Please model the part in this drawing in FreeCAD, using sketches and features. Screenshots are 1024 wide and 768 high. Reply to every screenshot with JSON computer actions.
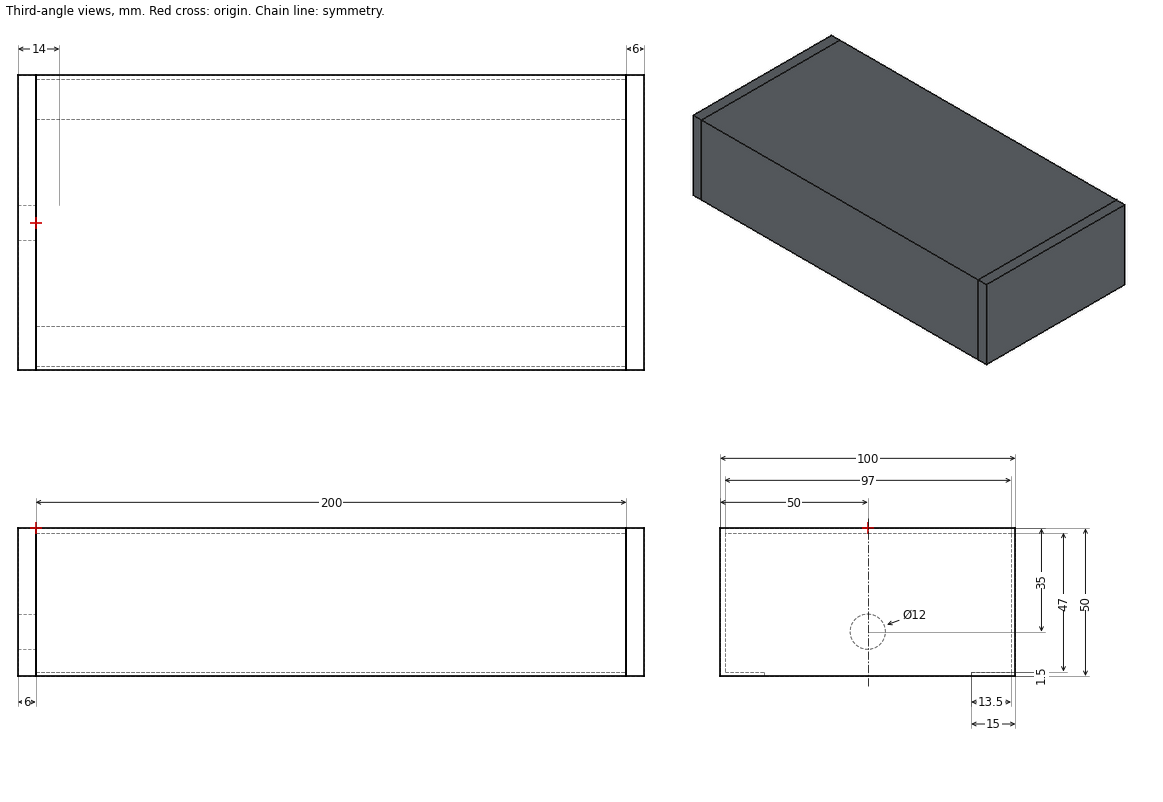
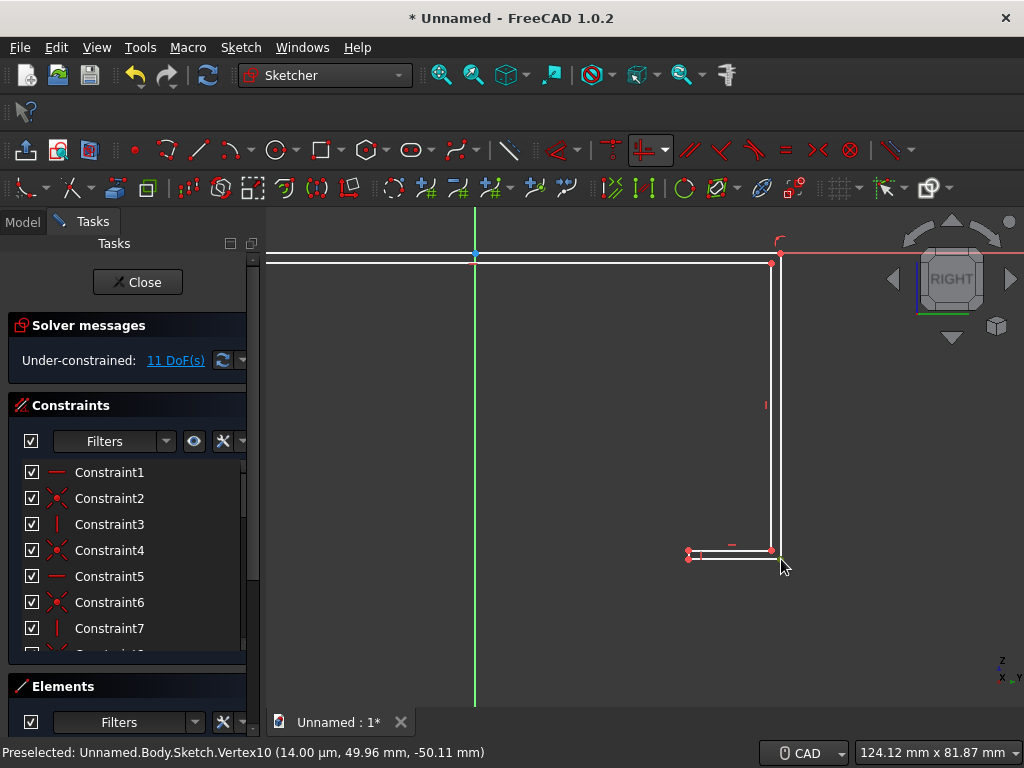
{"action": "scroll", "coordinate": [782, 560], "scroll_direction": "down", "scroll_amount": 2}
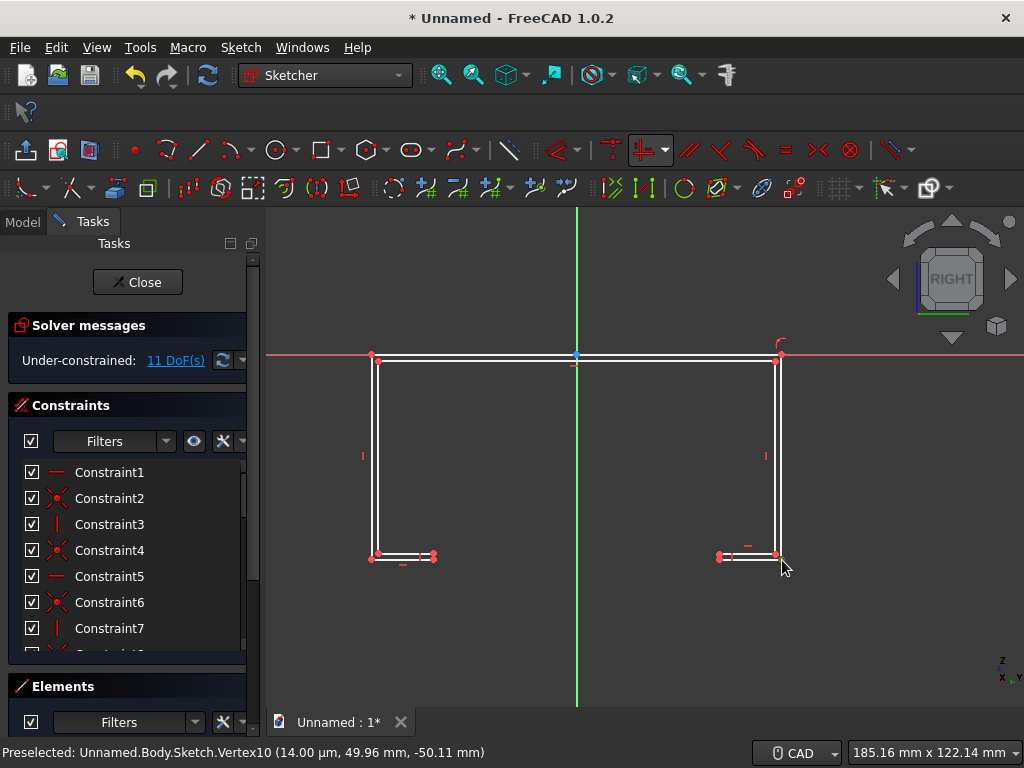
{"action": "scroll", "coordinate": [372, 560], "scroll_direction": "up", "scroll_amount": 2}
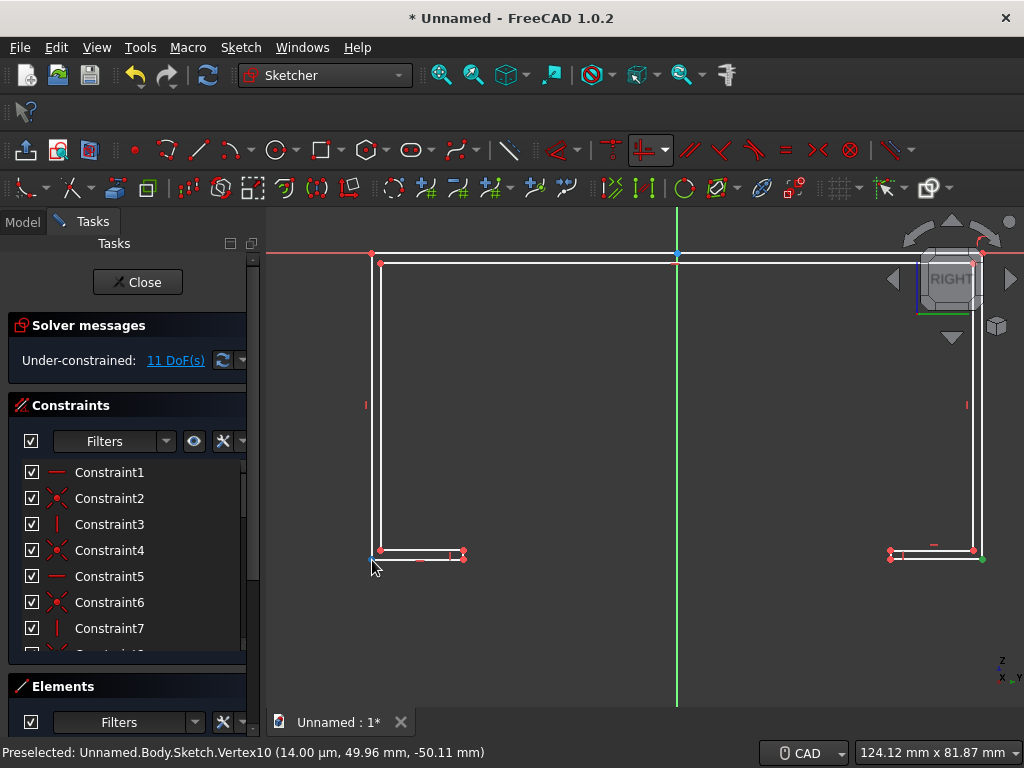
{"action": "left_click", "coordinate": [372, 560]}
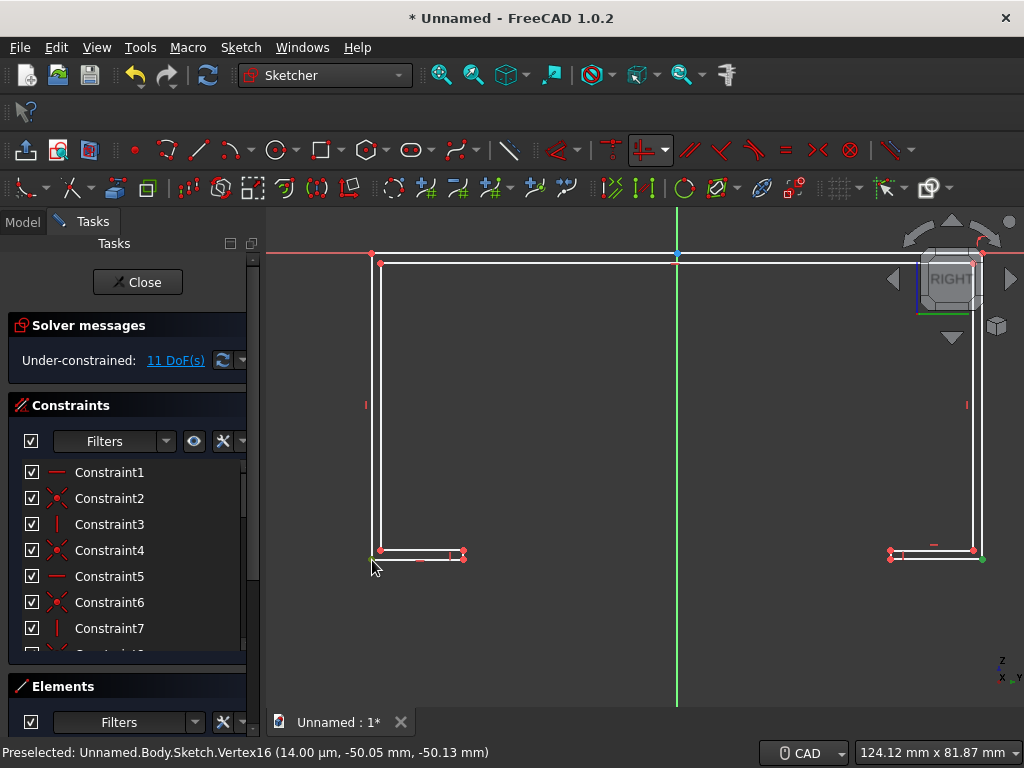
{"action": "left_click", "coordinate": [677, 647]}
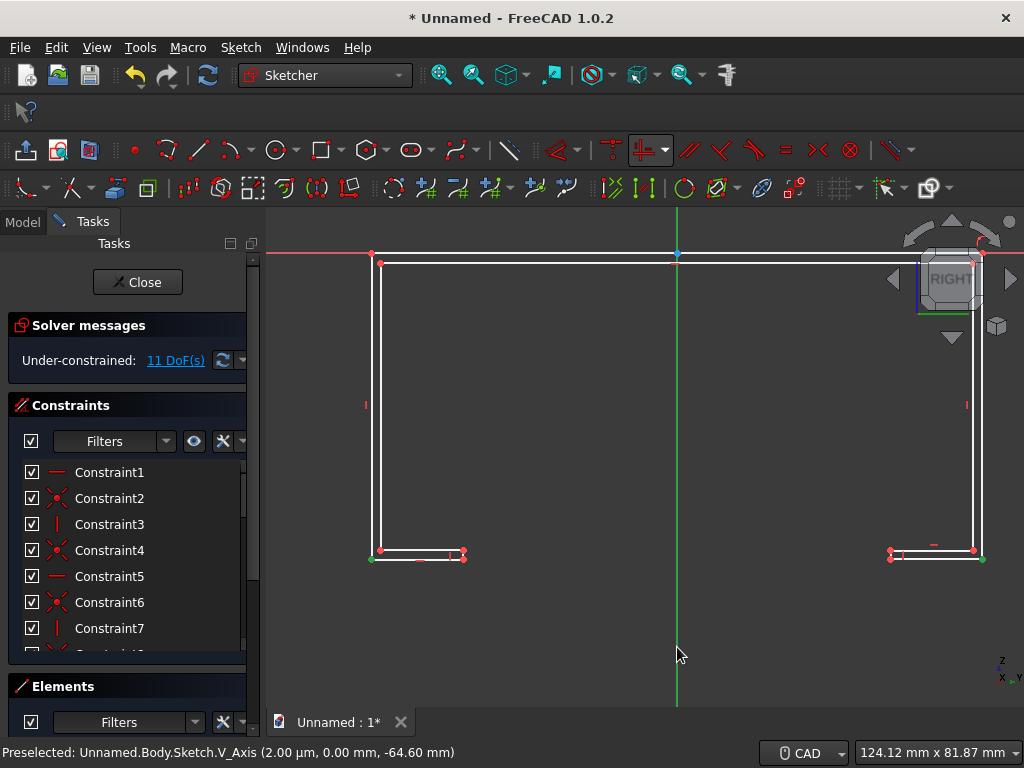
{"action": "key", "text": "s"}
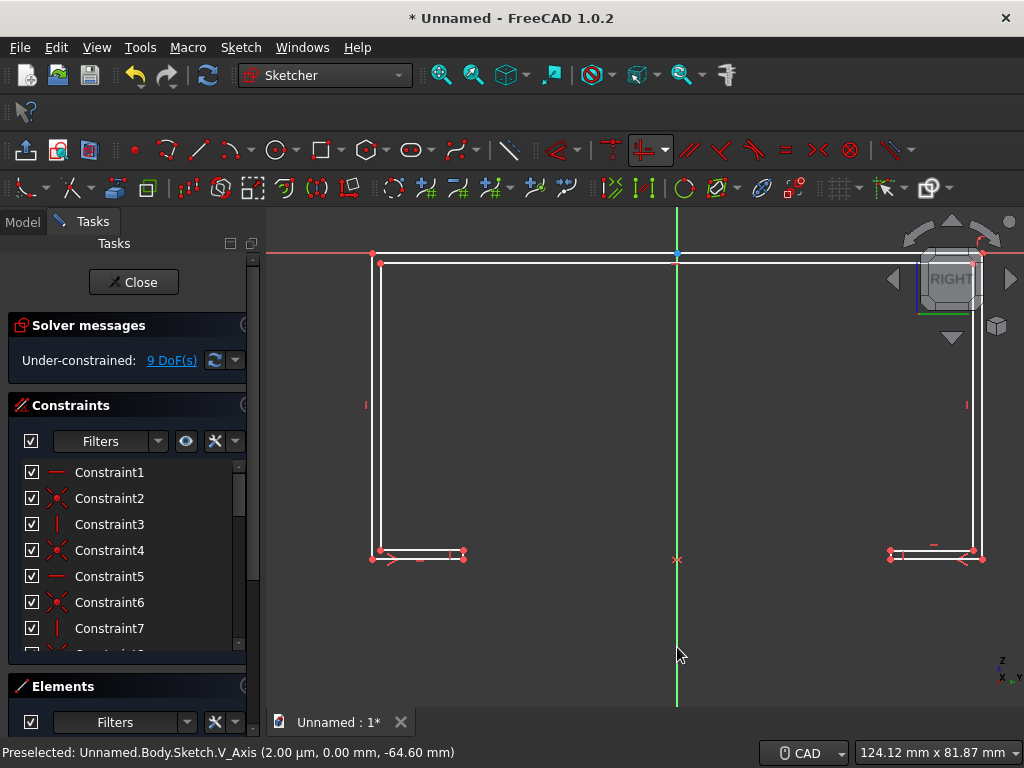
{"action": "scroll", "coordinate": [371, 560], "scroll_direction": "down", "scroll_amount": 2}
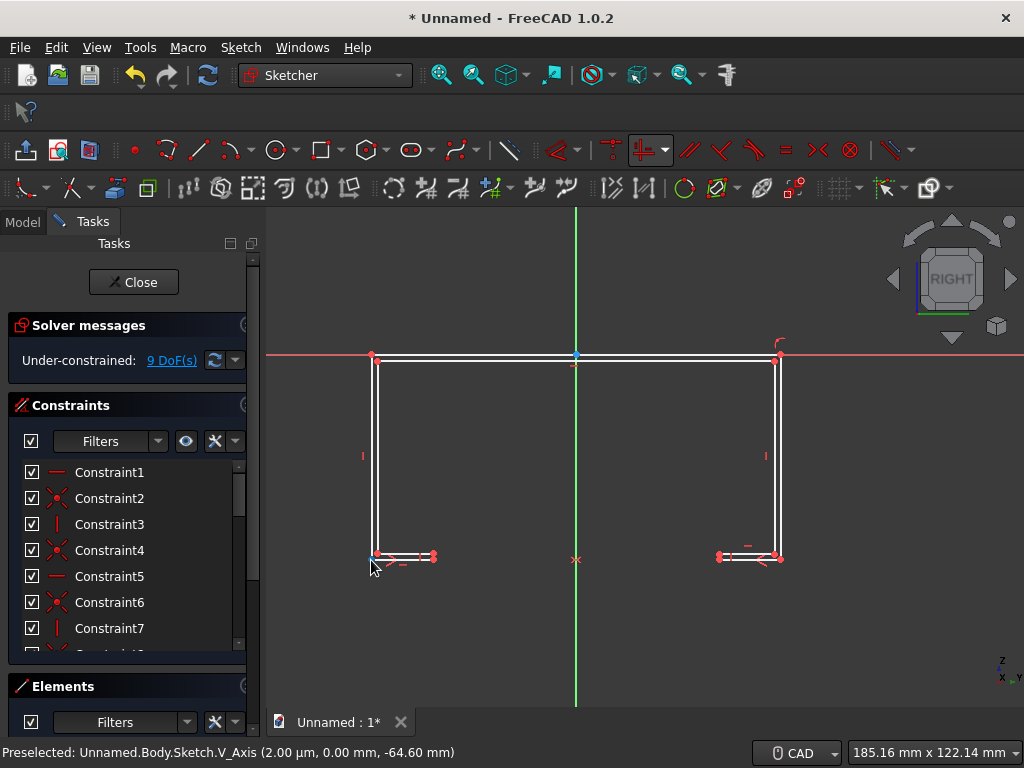
{"action": "scroll", "coordinate": [719, 554], "scroll_direction": "up", "scroll_amount": 4}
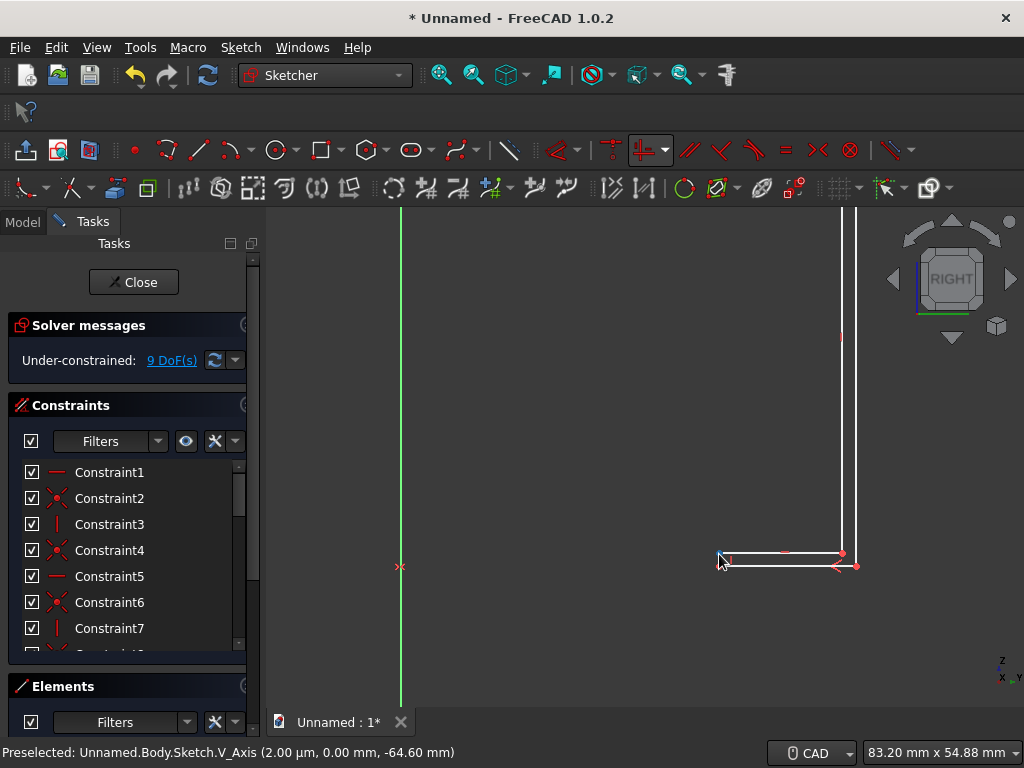
{"action": "left_click", "coordinate": [719, 553]}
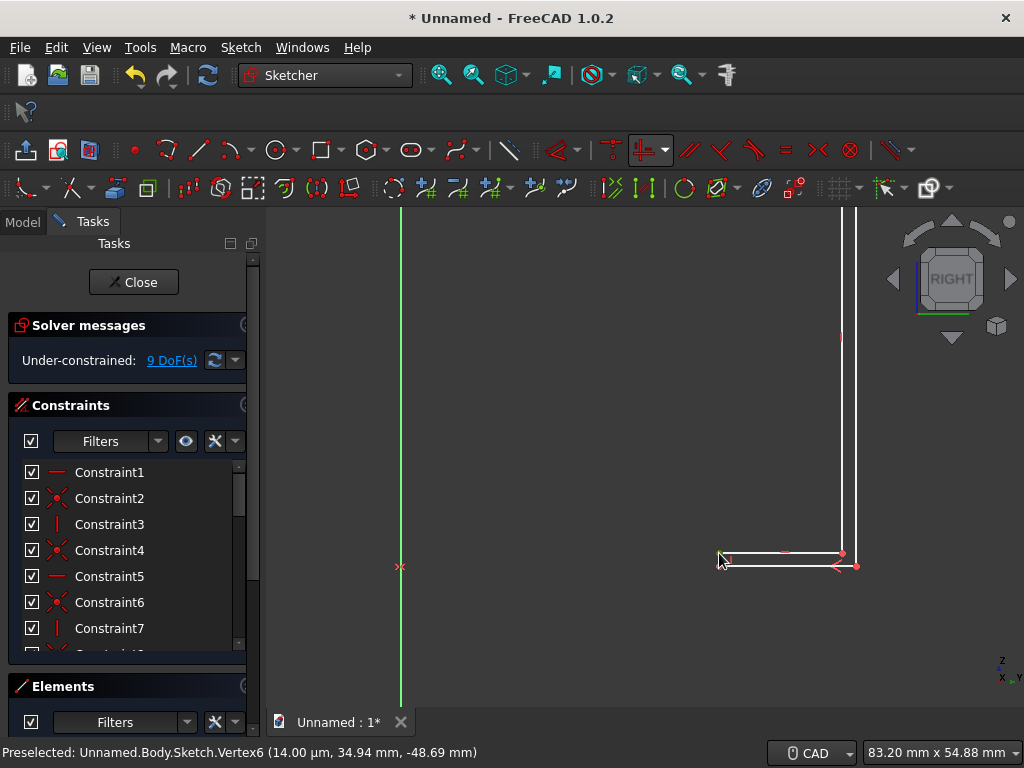
{"action": "scroll", "coordinate": [720, 554], "scroll_direction": "down", "scroll_amount": 4}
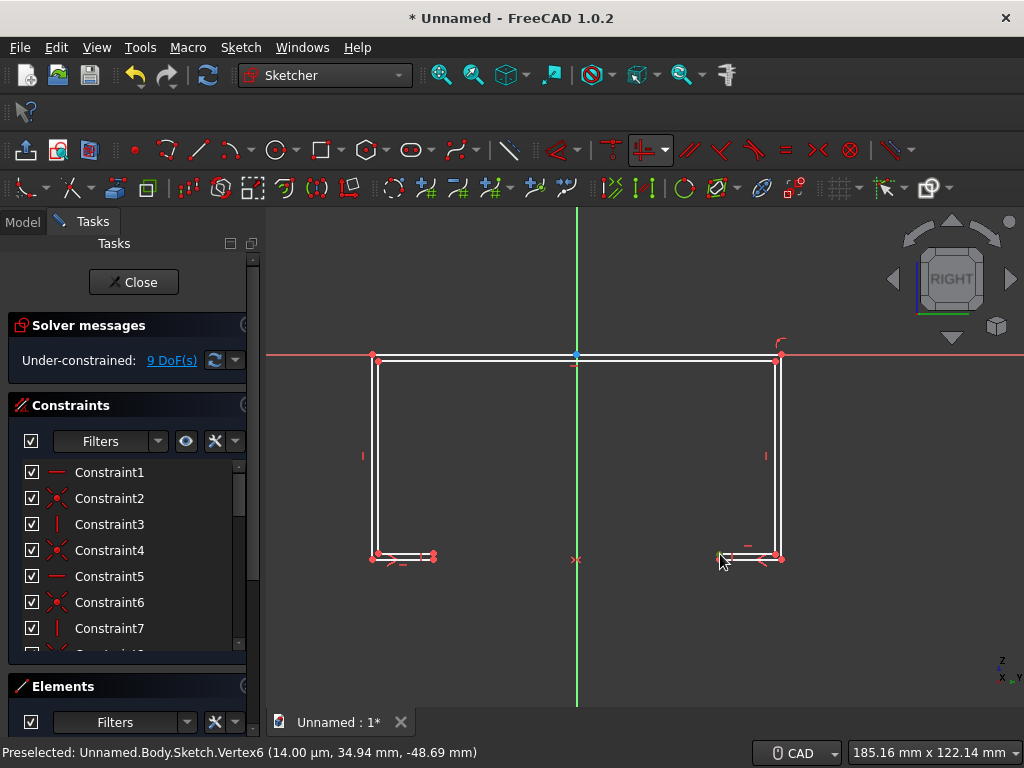
{"action": "scroll", "coordinate": [434, 554], "scroll_direction": "up", "scroll_amount": 4}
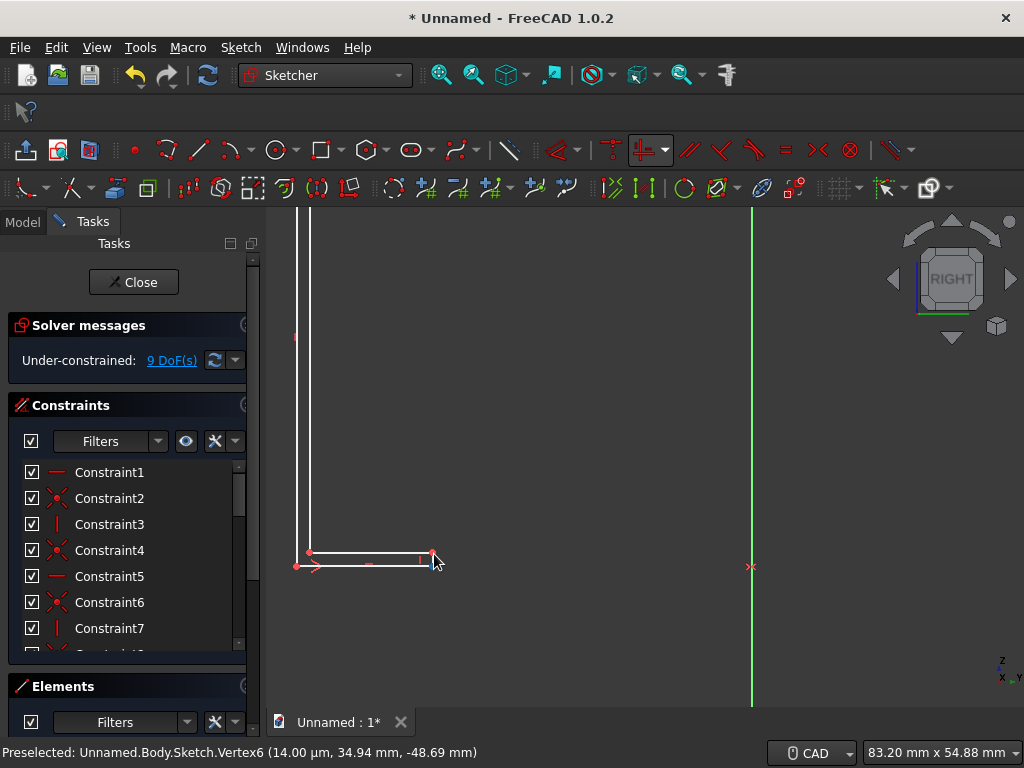
{"action": "left_click", "coordinate": [433, 553]}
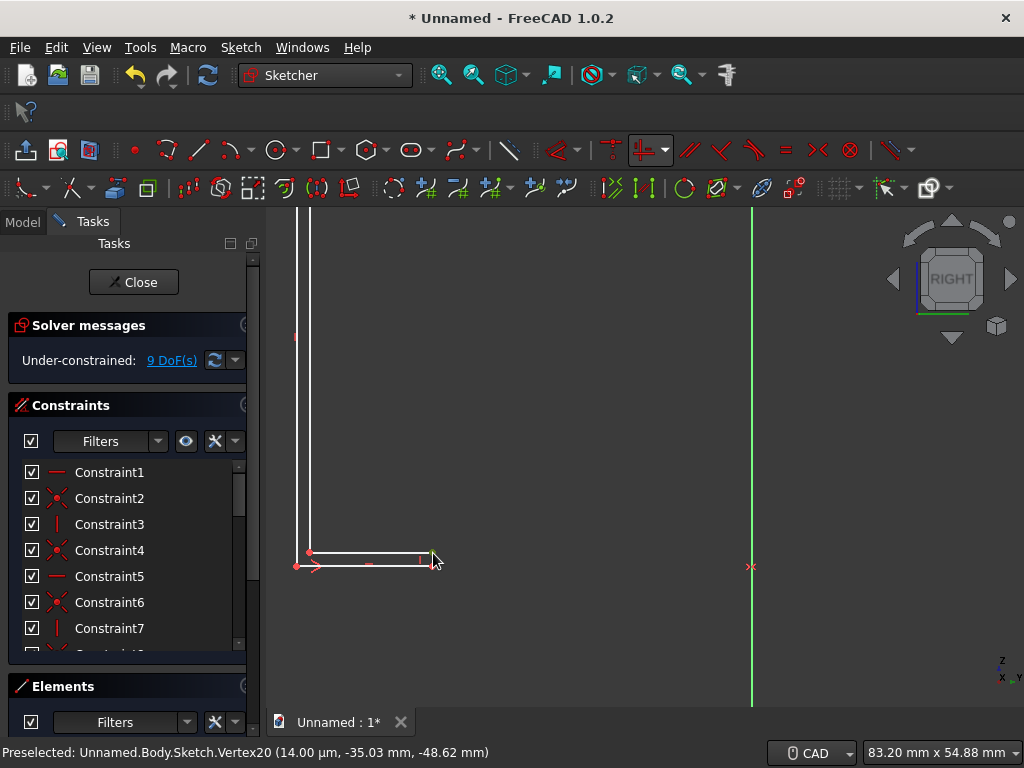
{"action": "left_click", "coordinate": [752, 647]}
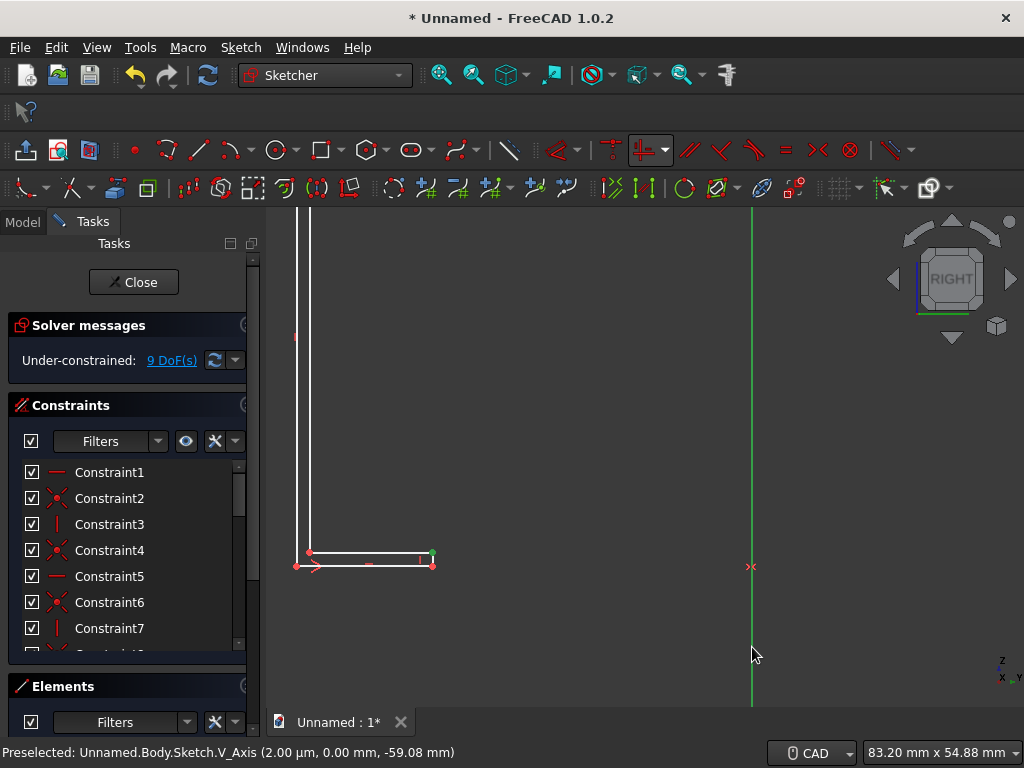
{"action": "key", "text": "s"}